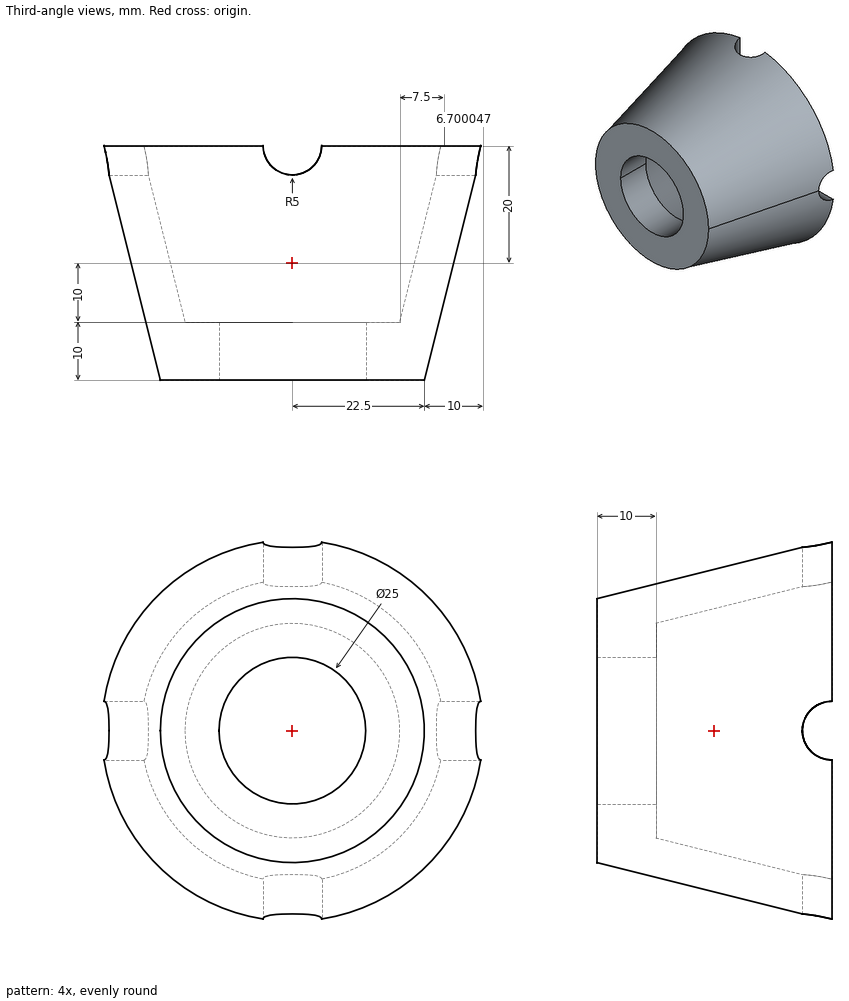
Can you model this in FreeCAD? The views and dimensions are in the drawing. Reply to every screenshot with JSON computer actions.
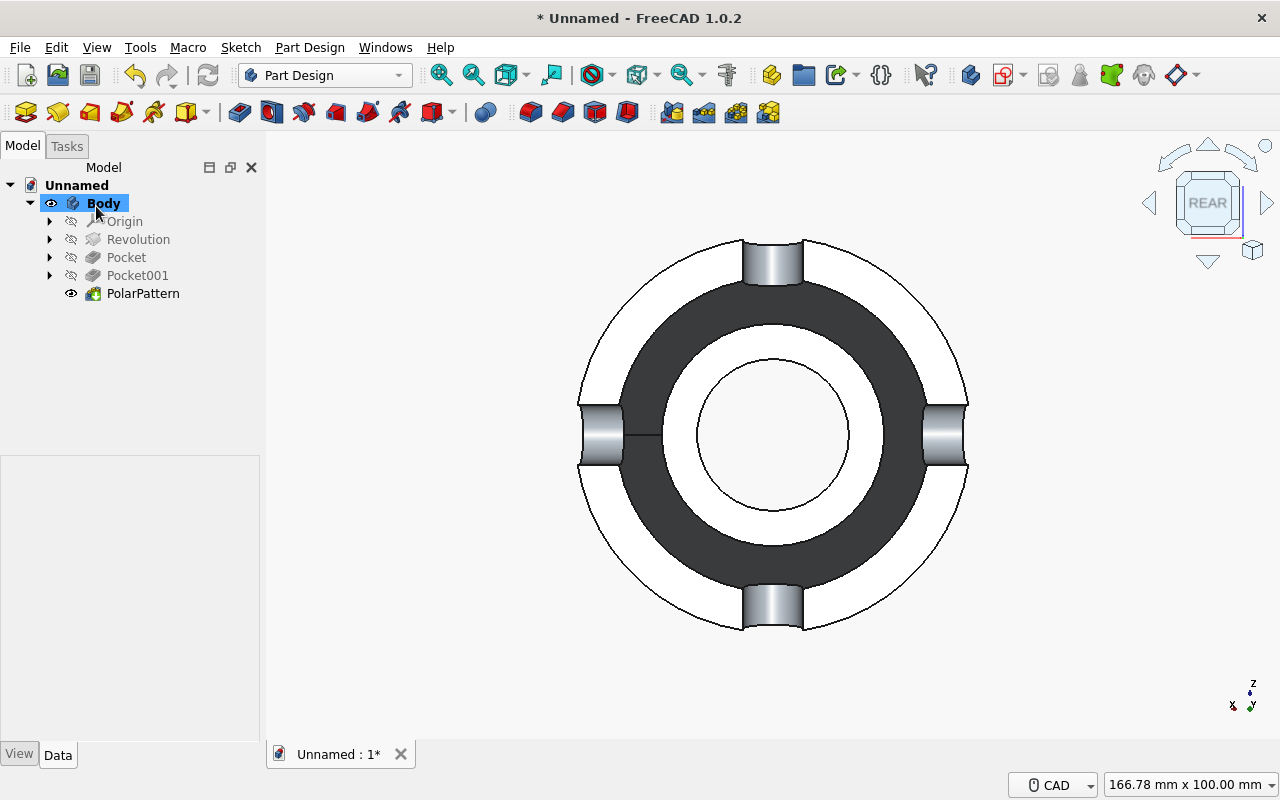
{"action": "key", "text": "0"}